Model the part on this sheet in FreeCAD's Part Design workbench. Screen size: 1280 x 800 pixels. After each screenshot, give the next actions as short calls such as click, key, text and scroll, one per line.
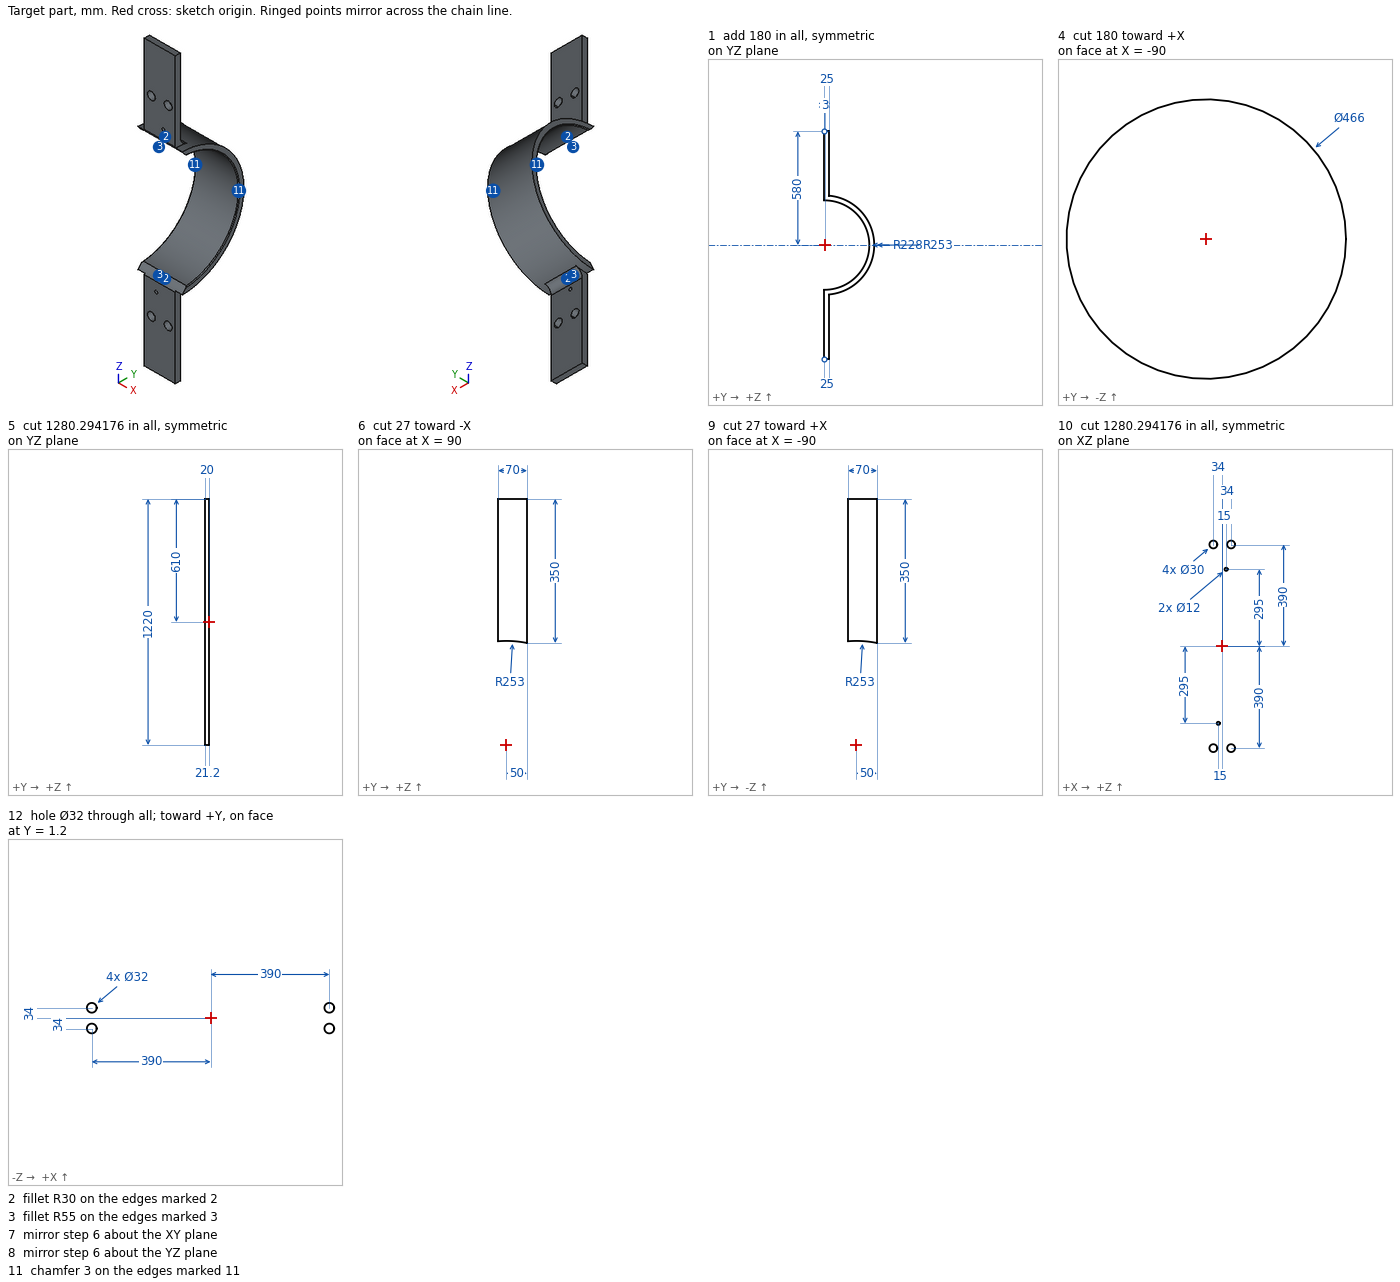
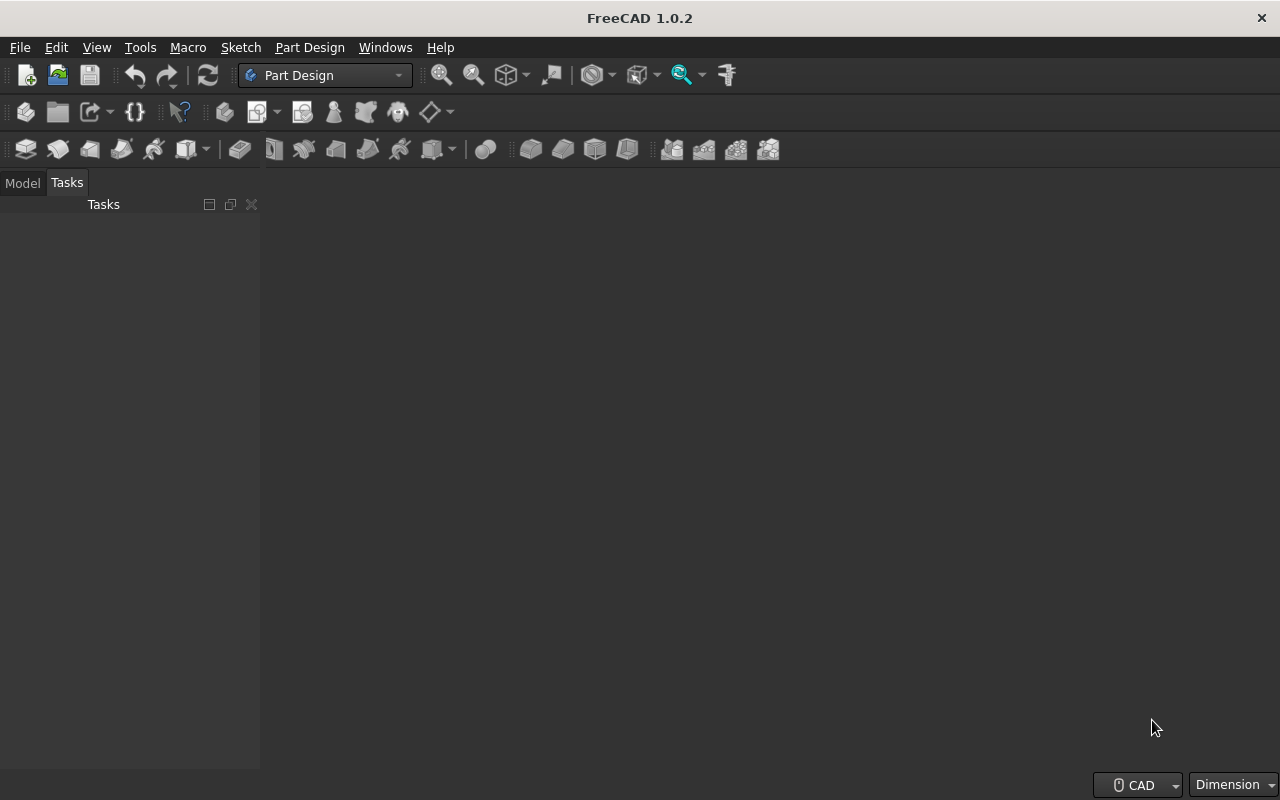
click(26, 76)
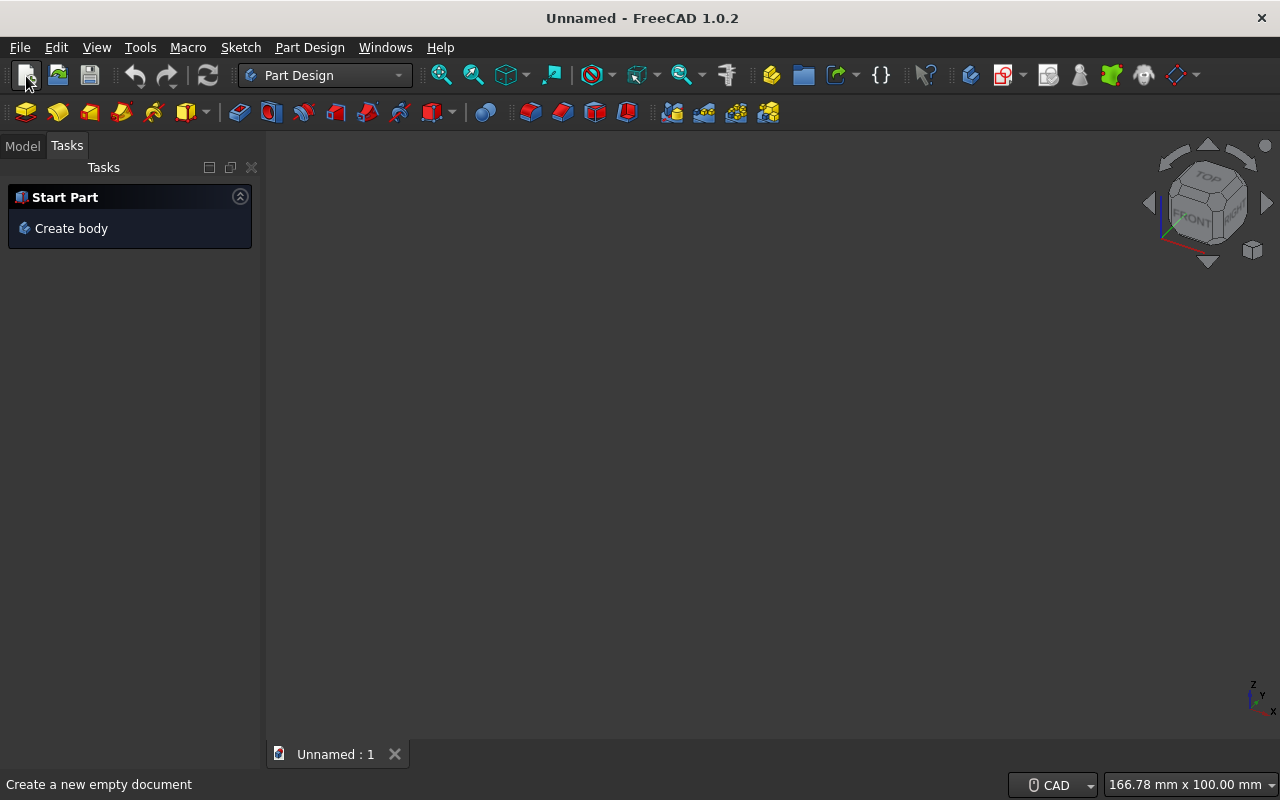
click(1004, 76)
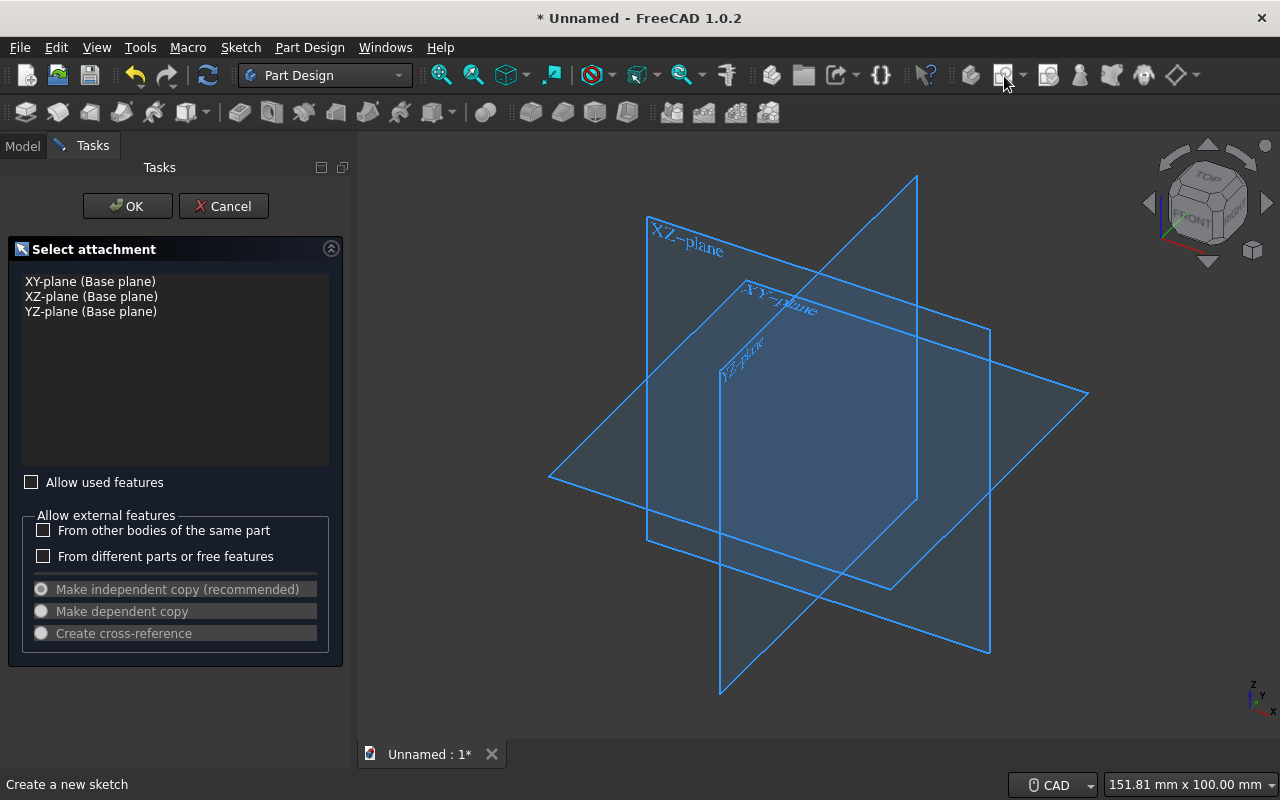
click(82, 312)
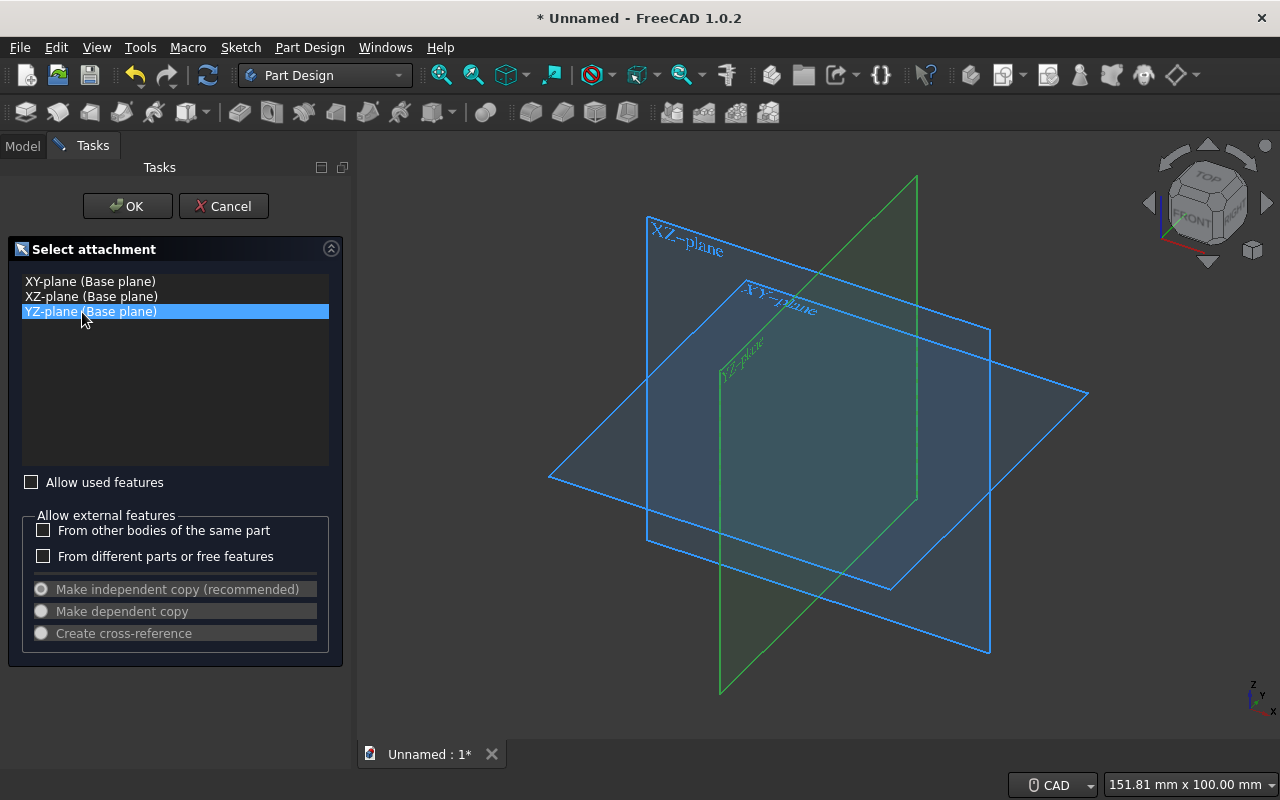
click(128, 206)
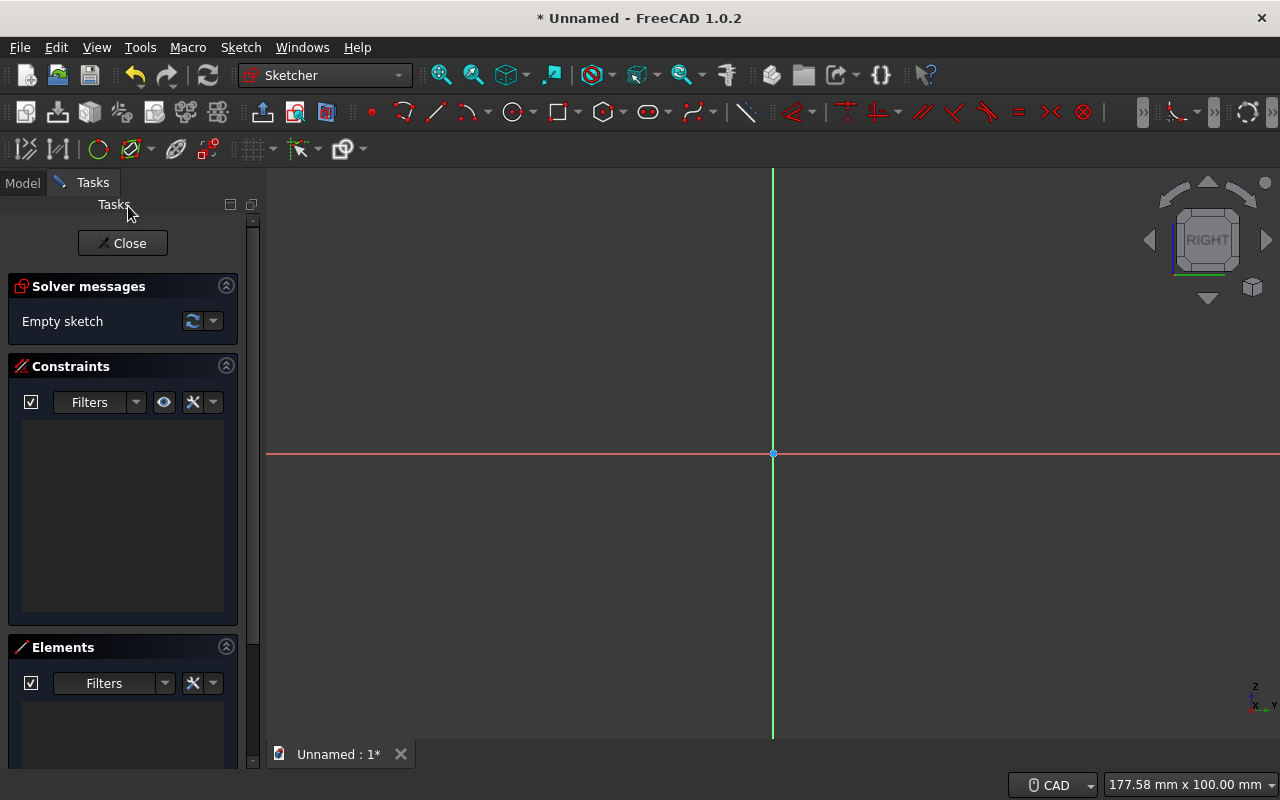
scroll(664, 454, down, 15)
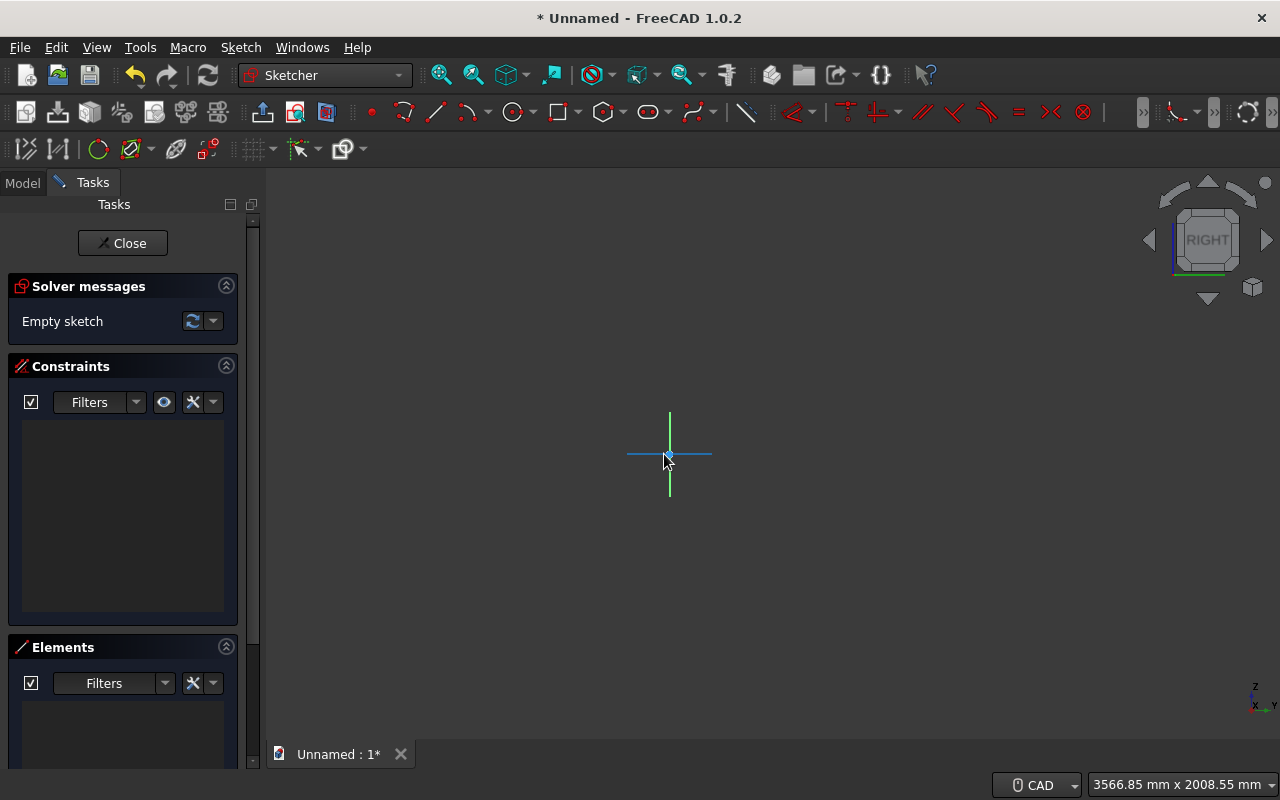
click(404, 112)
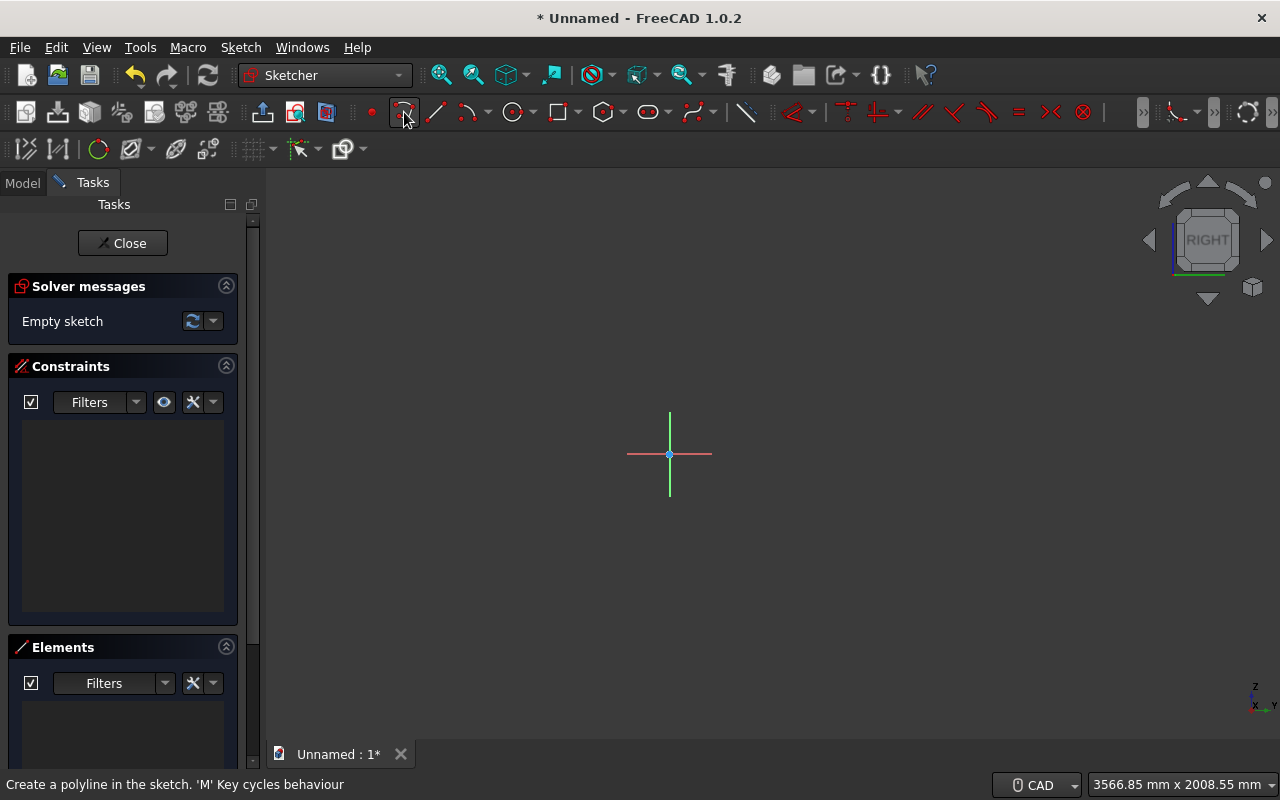
scroll(676, 383, up, 5)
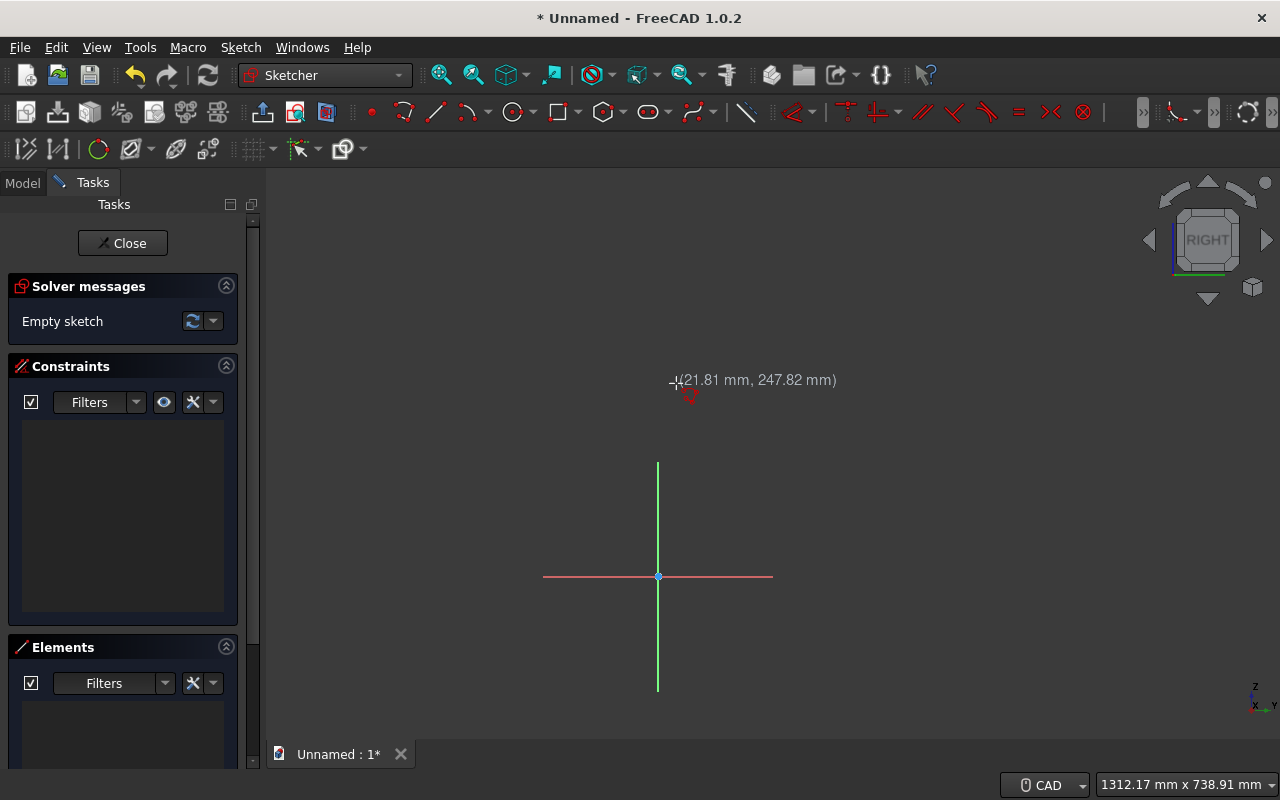
click(675, 382)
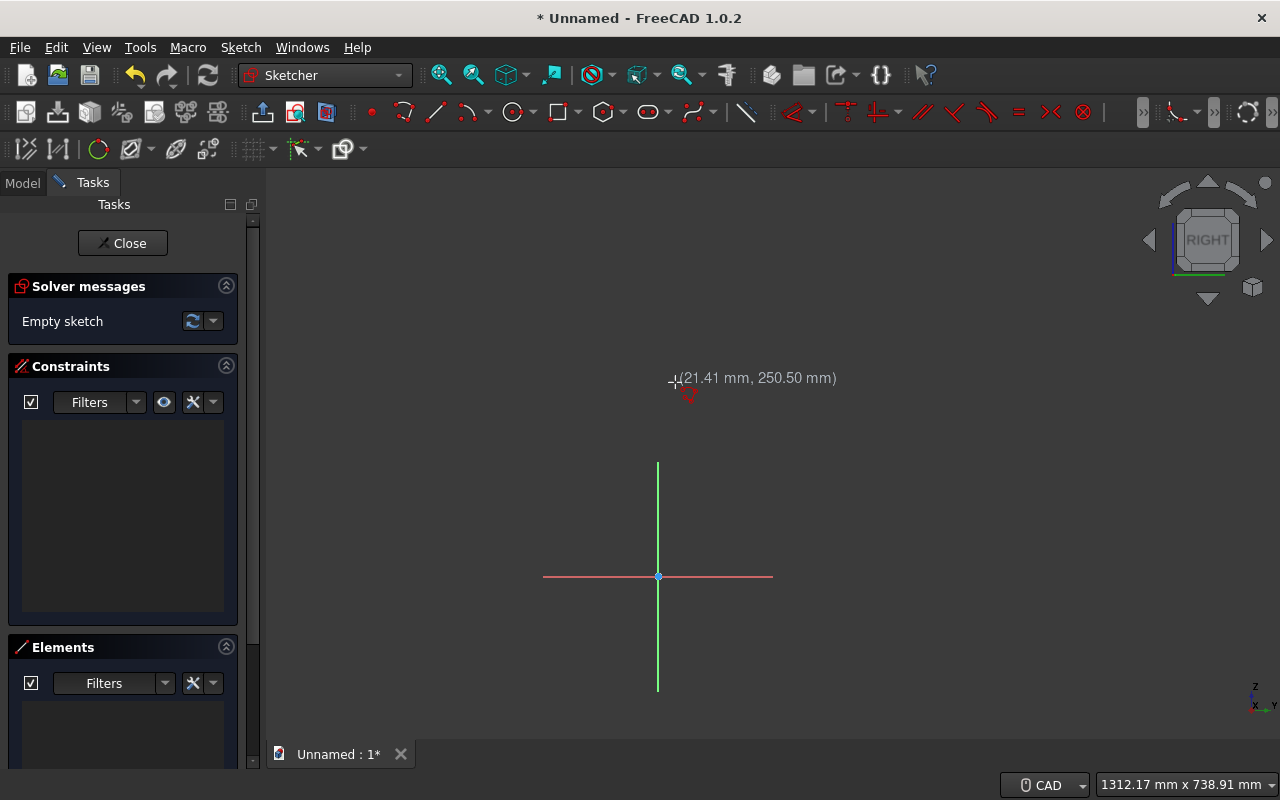
scroll(675, 382, down, 5)